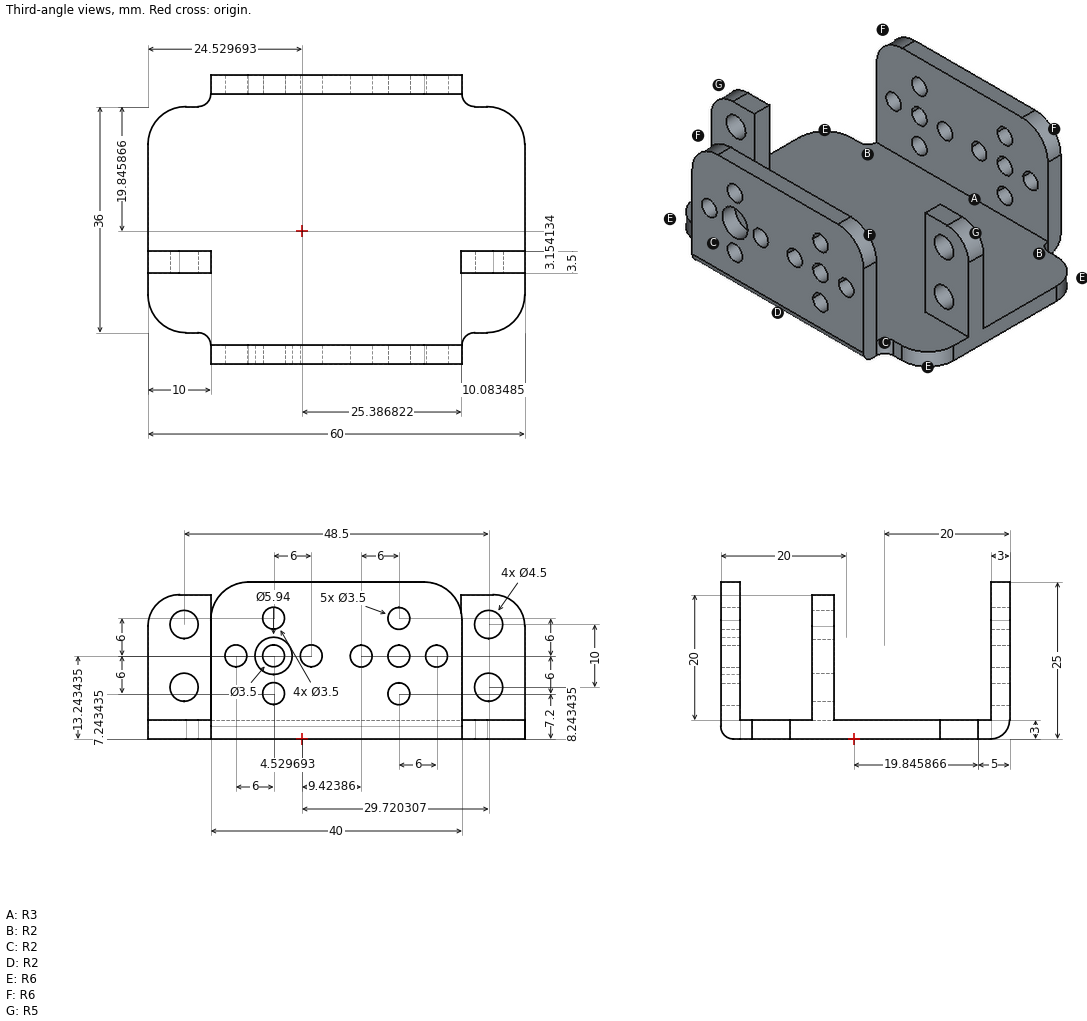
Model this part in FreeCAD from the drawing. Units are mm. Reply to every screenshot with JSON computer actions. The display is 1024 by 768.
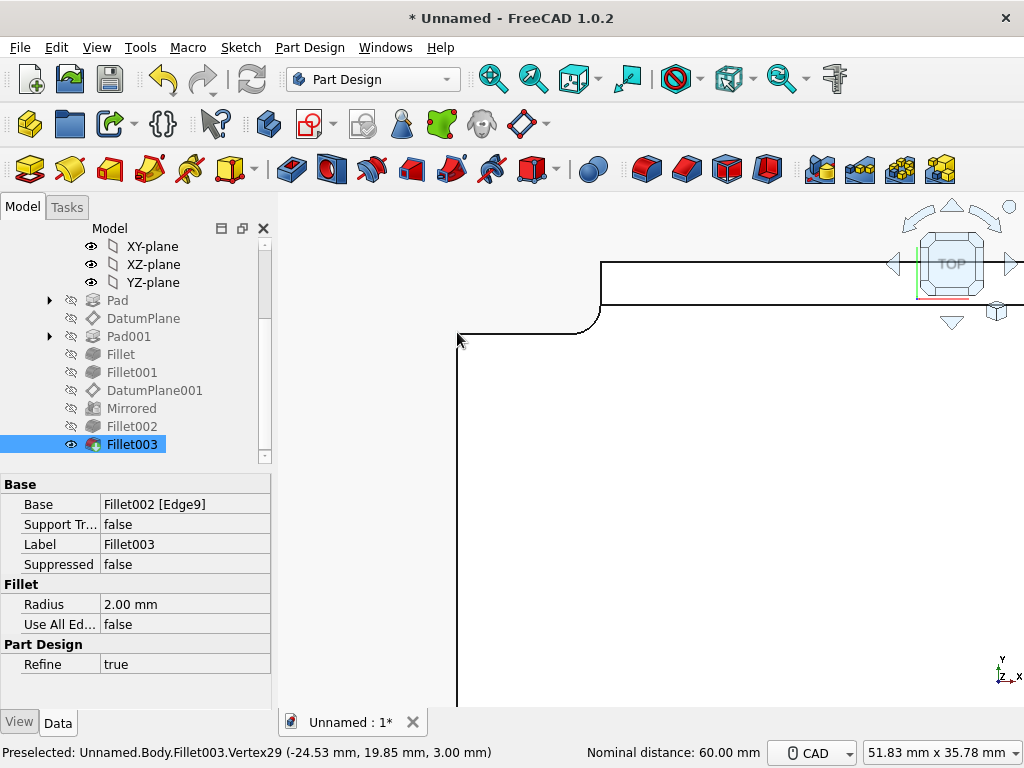
{"action": "left_click", "coordinate": [494, 80]}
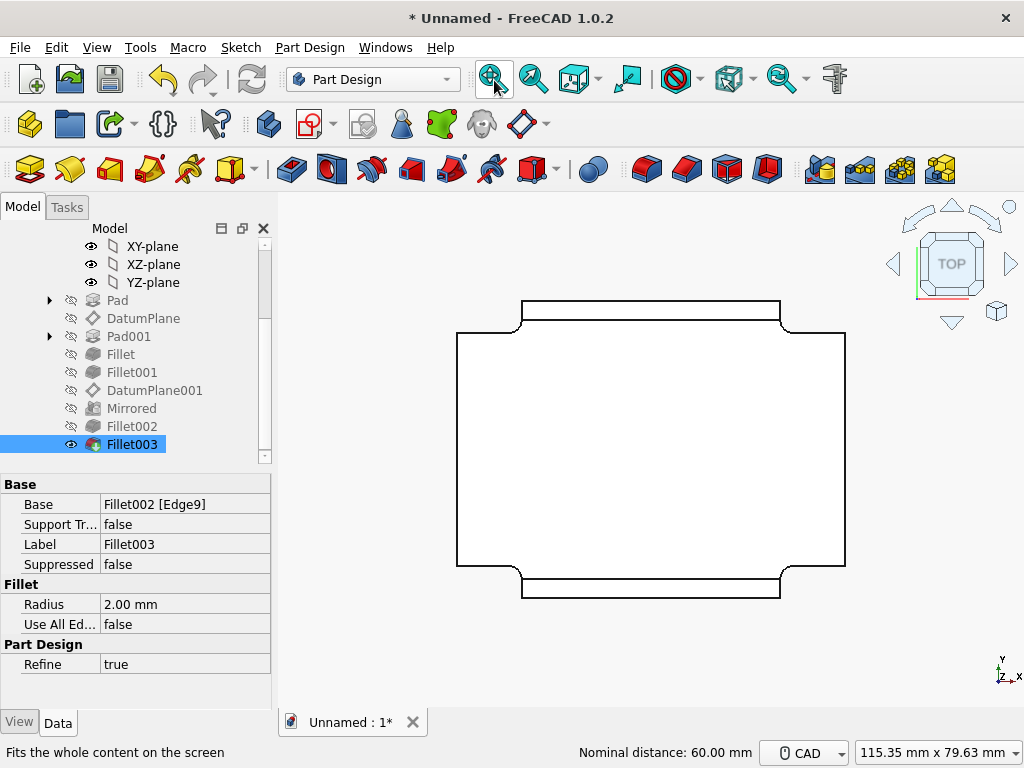
{"action": "key", "text": "1"}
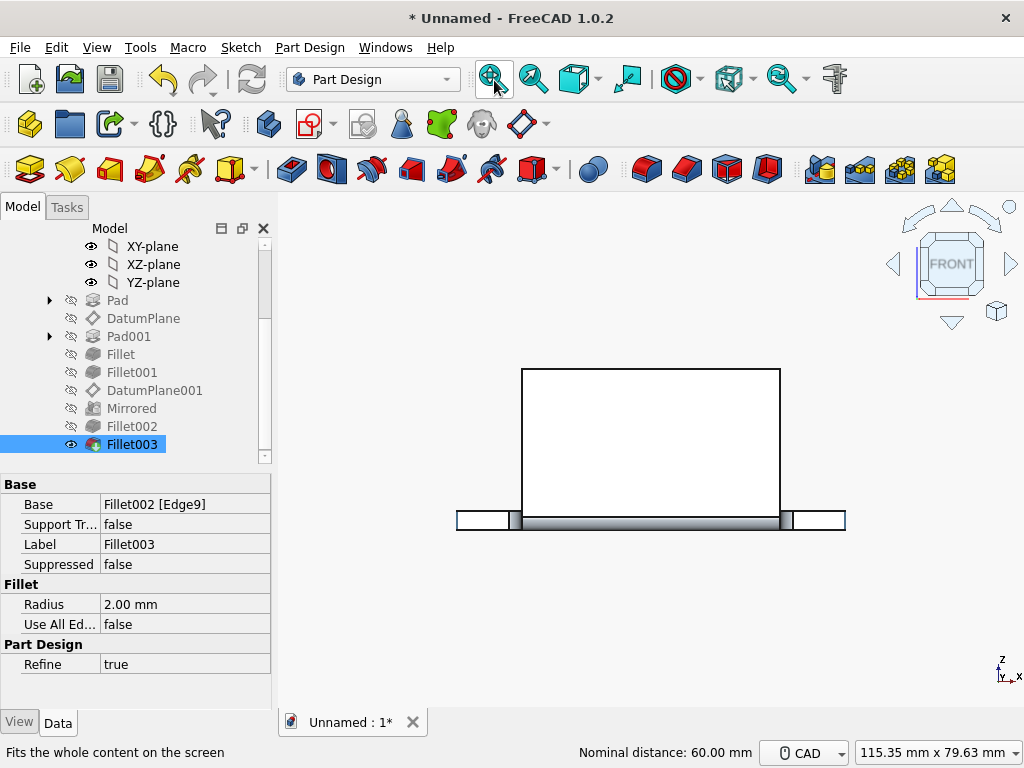
{"action": "scroll", "coordinate": [457, 520], "scroll_direction": "up", "scroll_amount": 4}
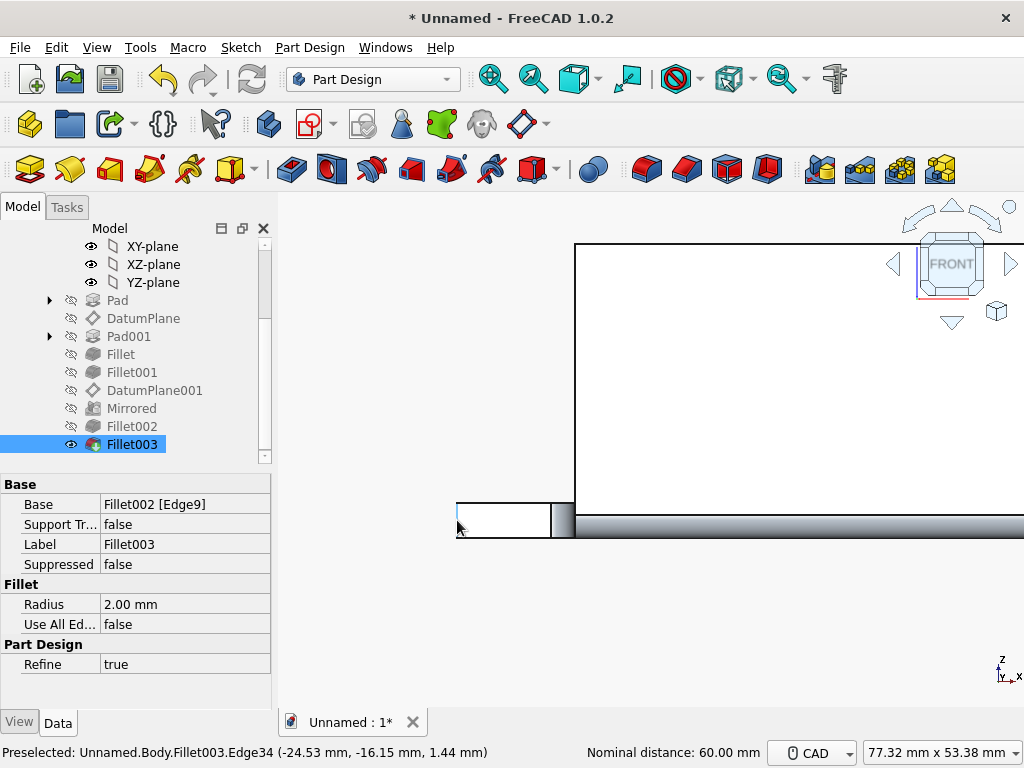
{"action": "left_click", "coordinate": [494, 80]}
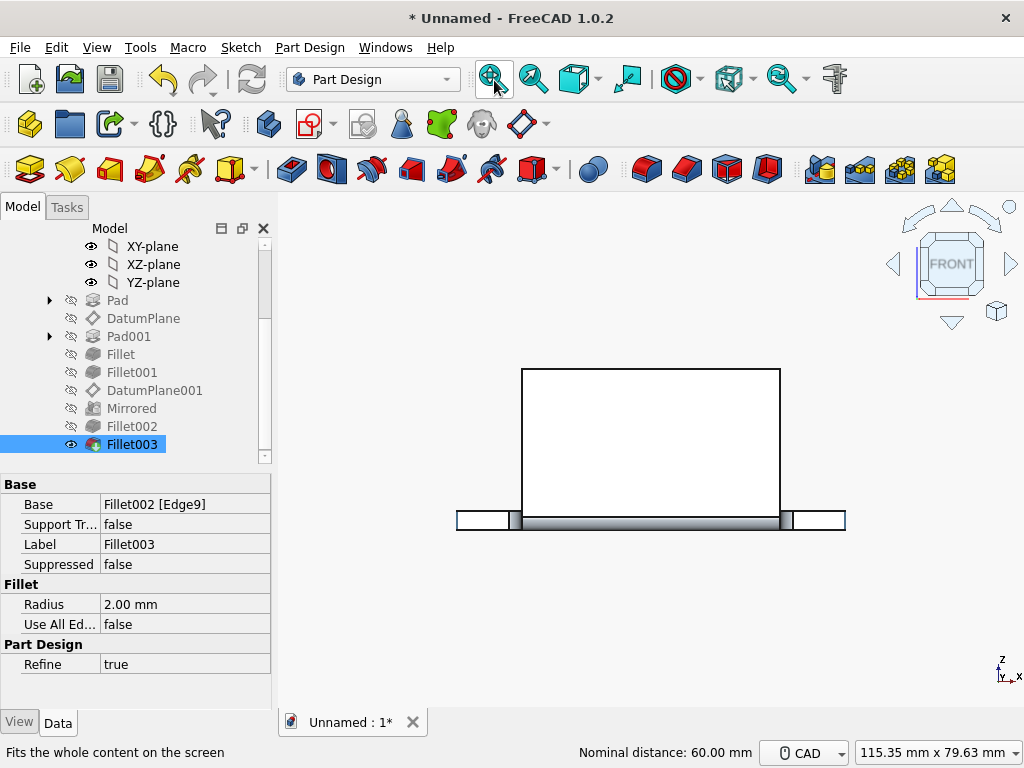
{"action": "key", "text": "3"}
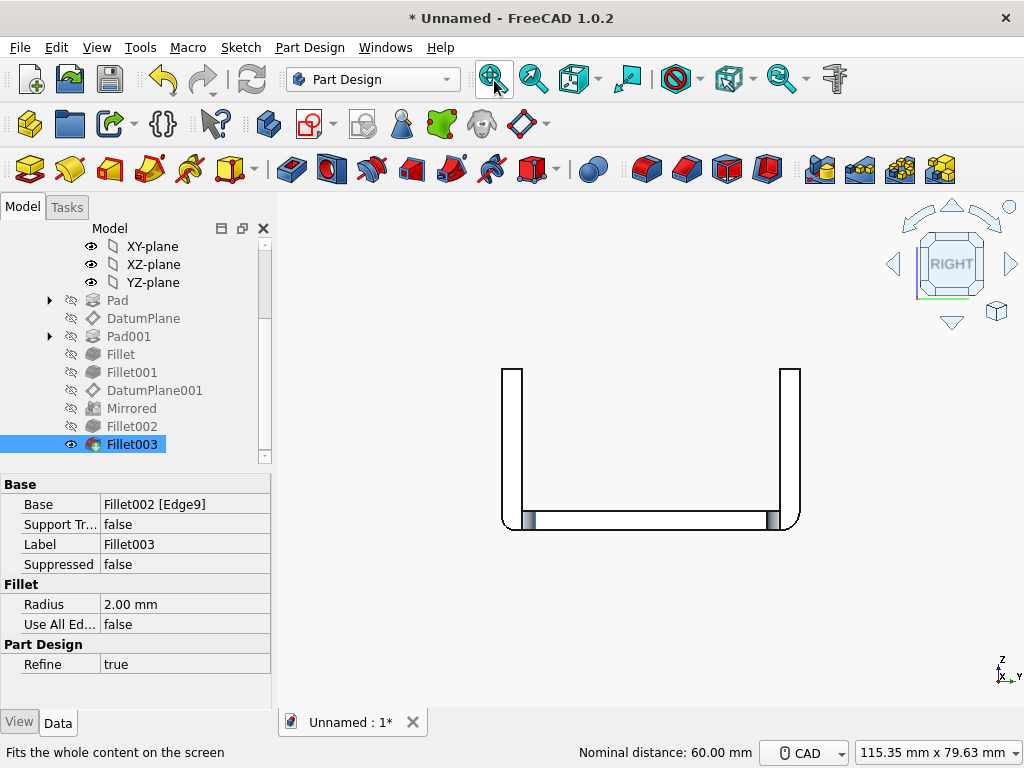
{"action": "left_click", "coordinate": [494, 80]}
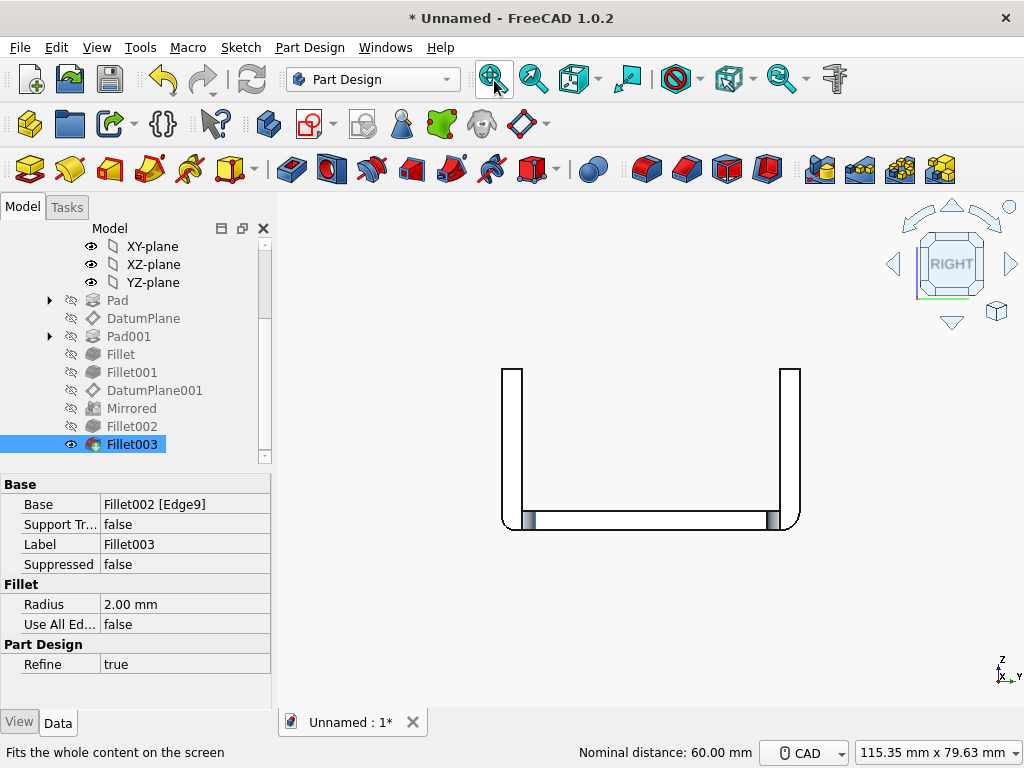
{"action": "left_click", "coordinate": [767, 520], "text": "ctrl"}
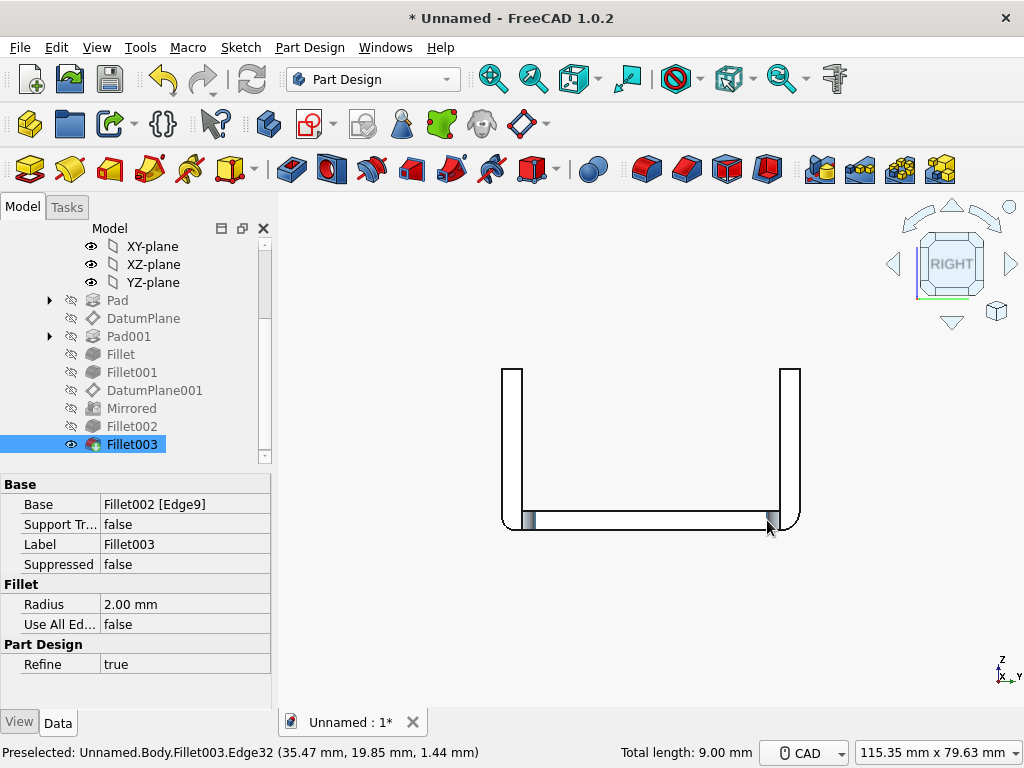
{"action": "scroll", "coordinate": [767, 520], "scroll_direction": "up", "scroll_amount": 4}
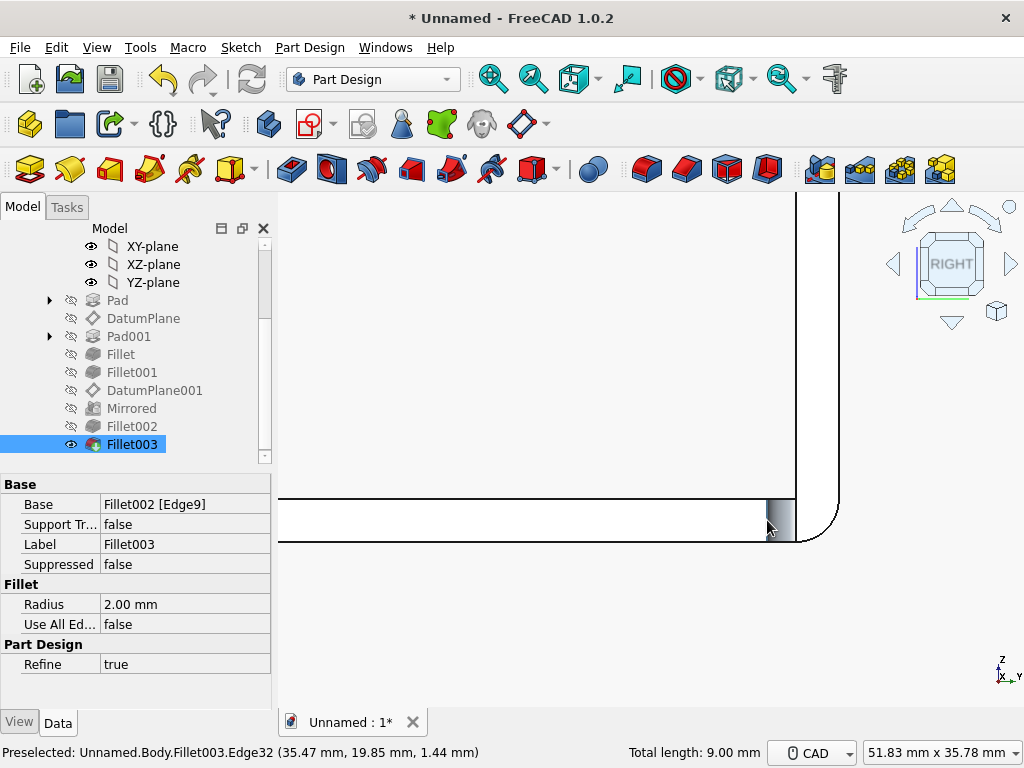
{"action": "left_click", "coordinate": [494, 80]}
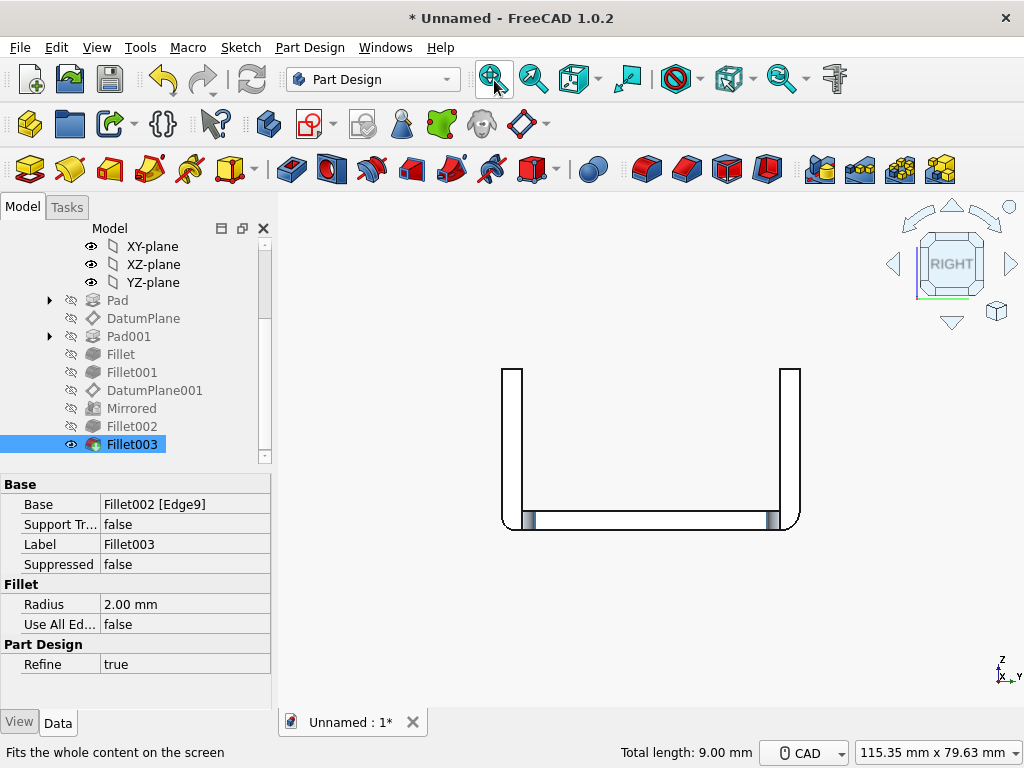
{"action": "key", "text": "5"}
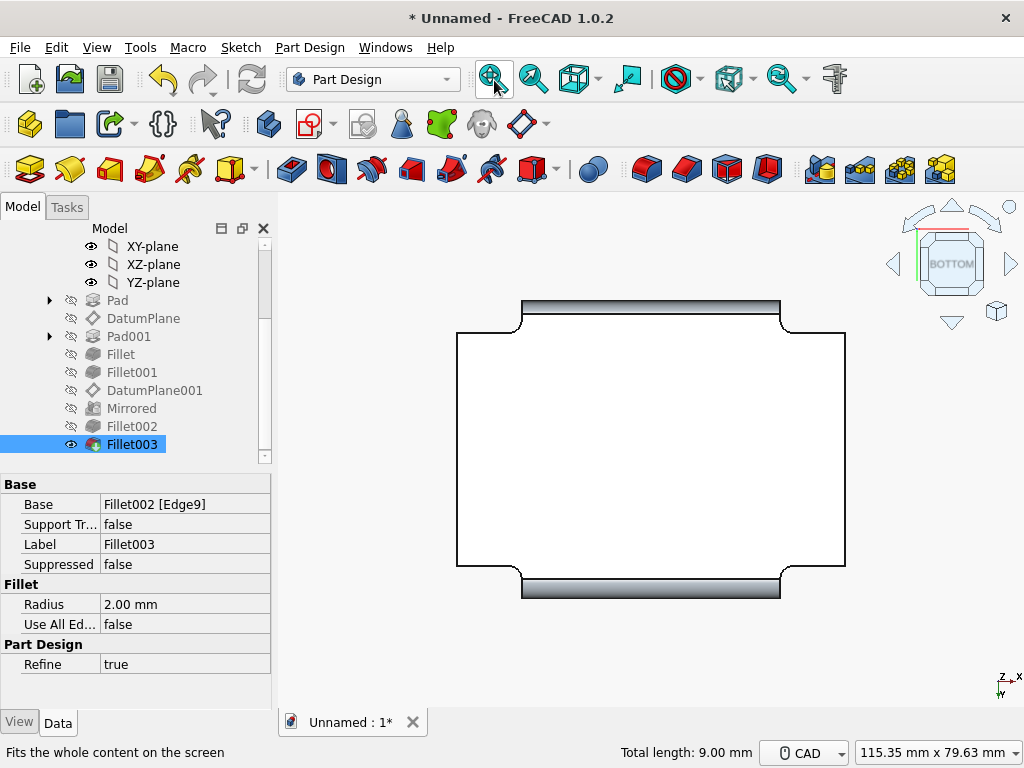
{"action": "scroll", "coordinate": [457, 565], "scroll_direction": "up", "scroll_amount": 4}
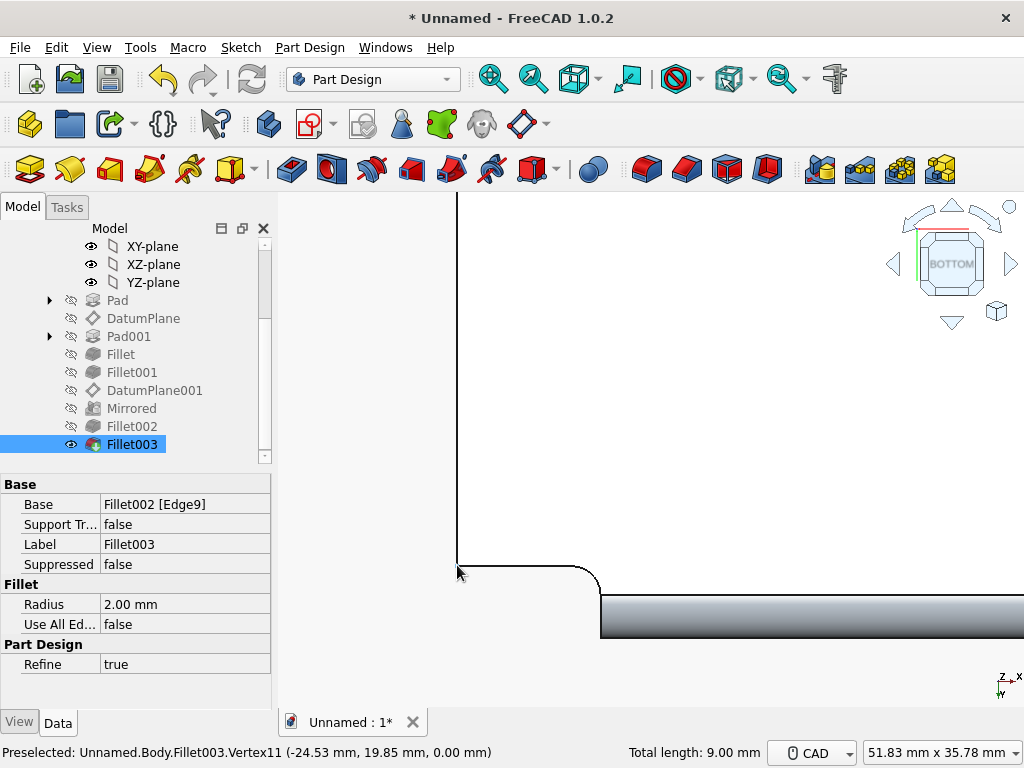
{"action": "left_click", "coordinate": [494, 80]}